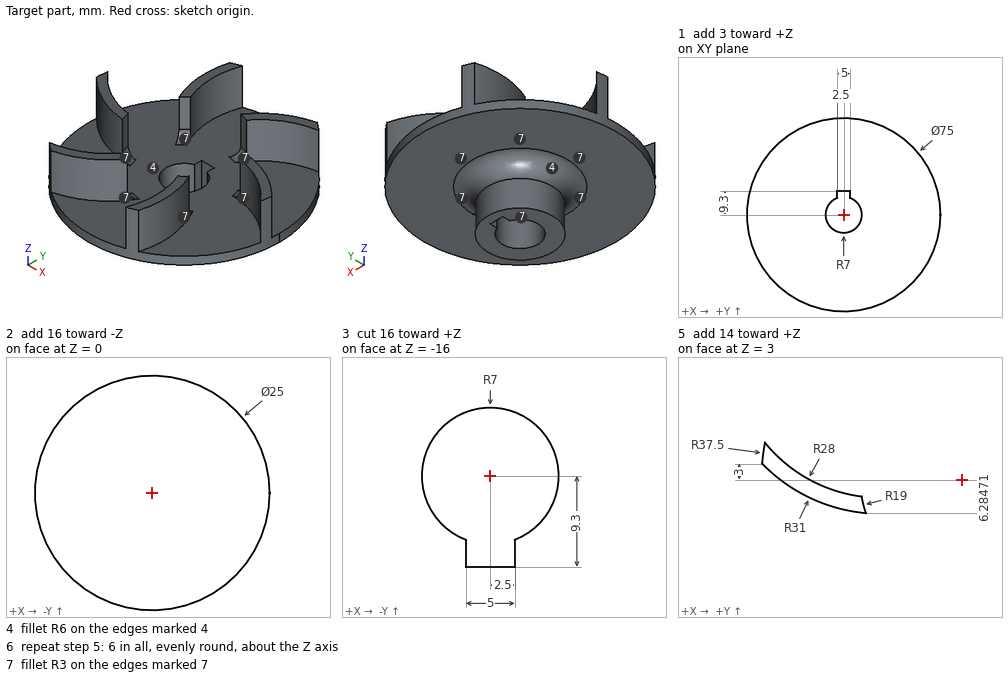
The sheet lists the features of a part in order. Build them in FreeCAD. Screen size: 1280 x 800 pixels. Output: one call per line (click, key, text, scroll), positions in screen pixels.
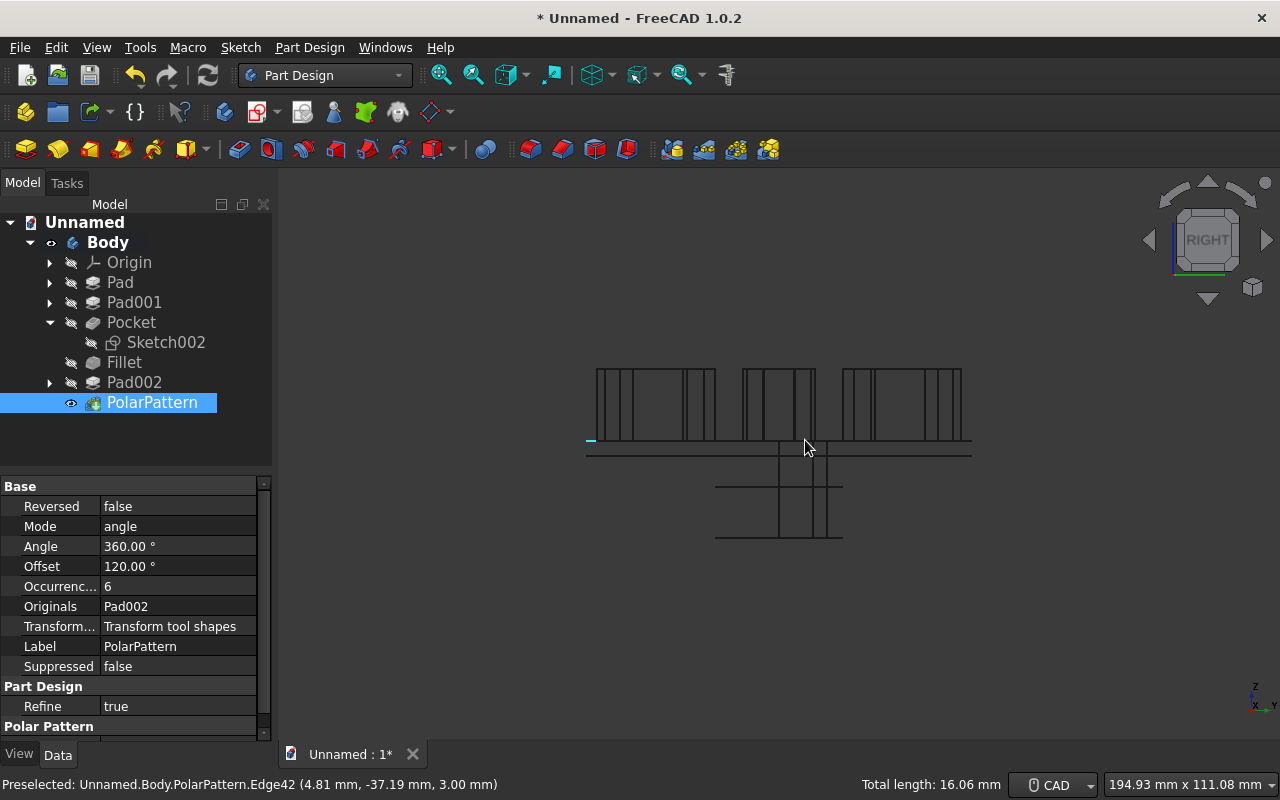
scroll(873, 440, up, 5)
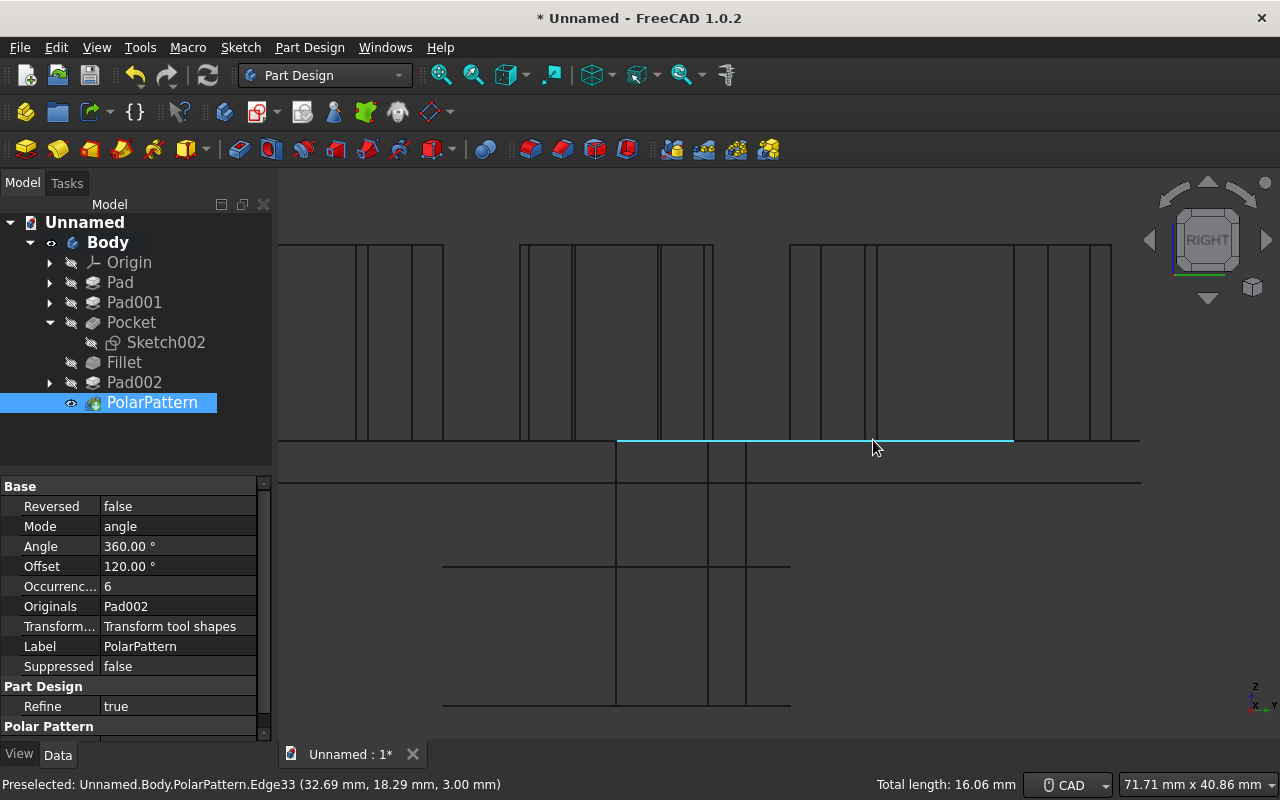
key(v)
key(f)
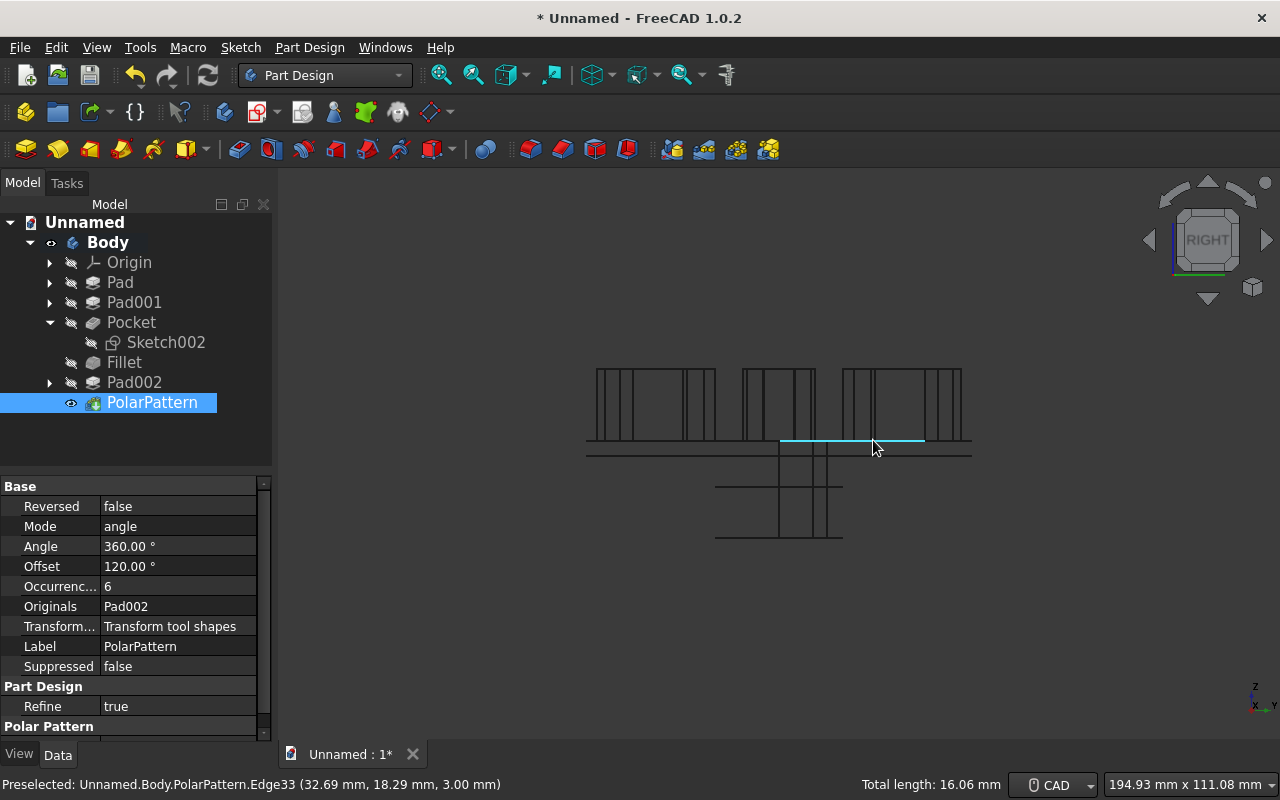
key(5)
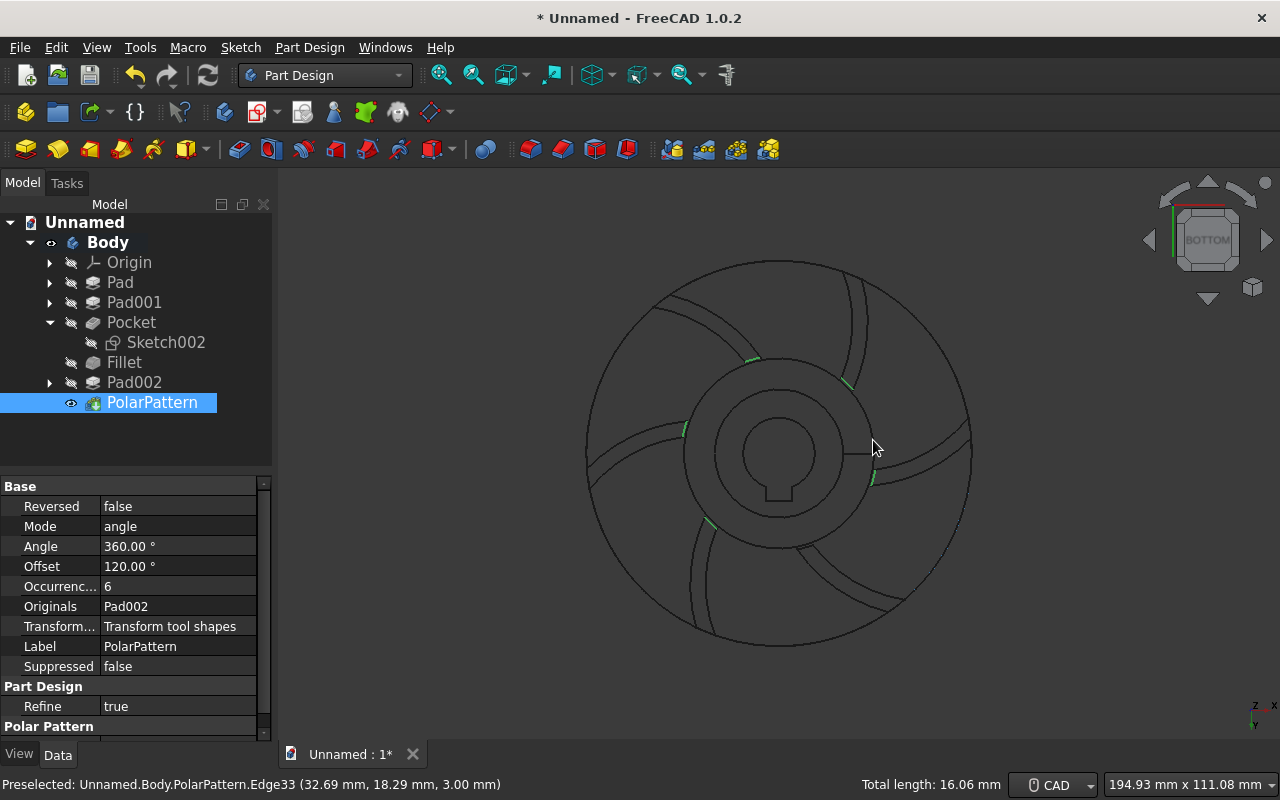
scroll(805, 547, up, 5)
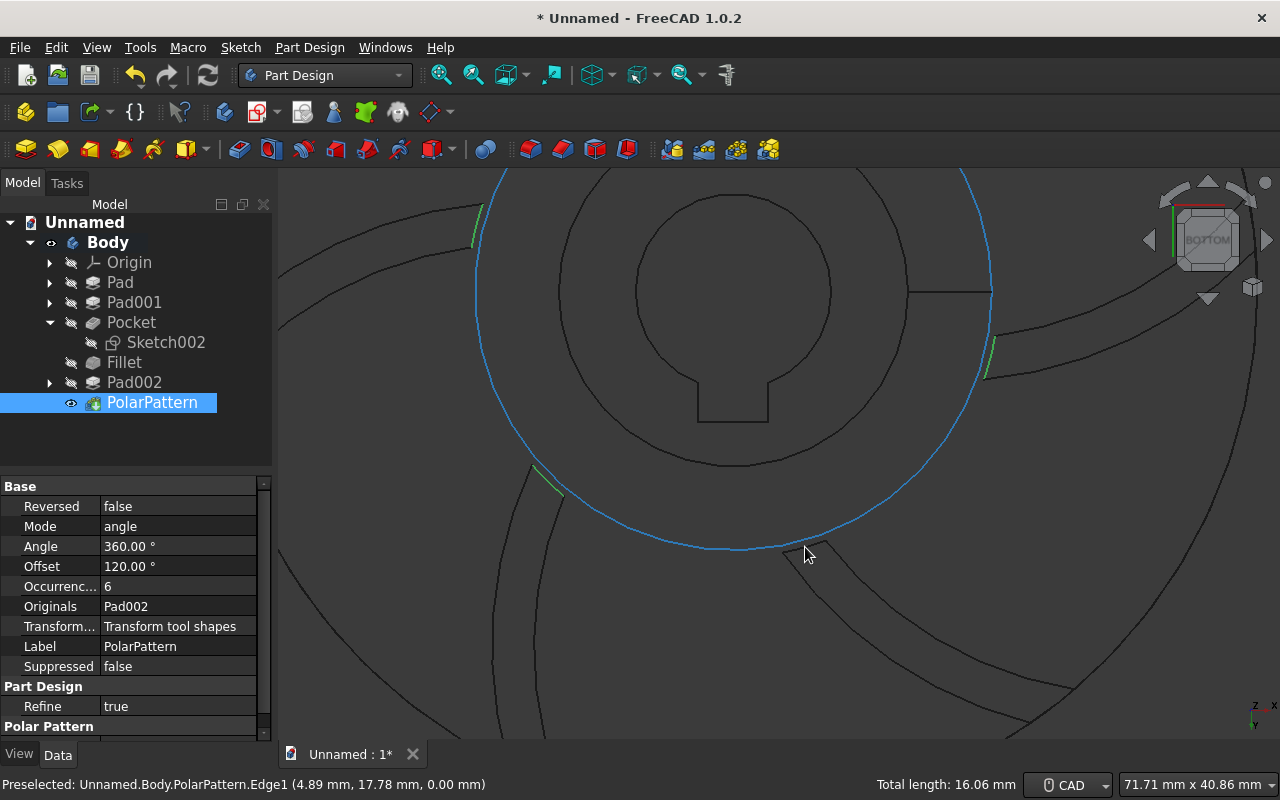
click(804, 546, ctrl)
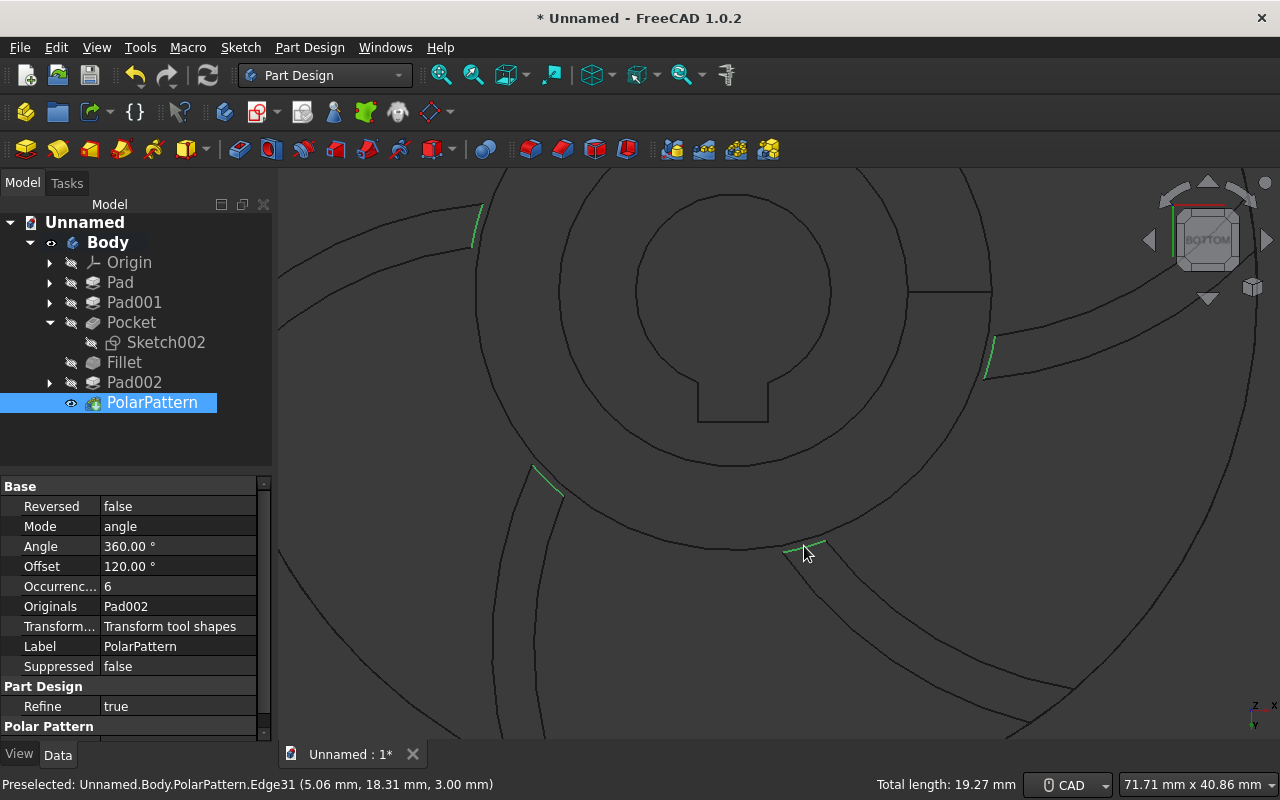
key(v)
key(1)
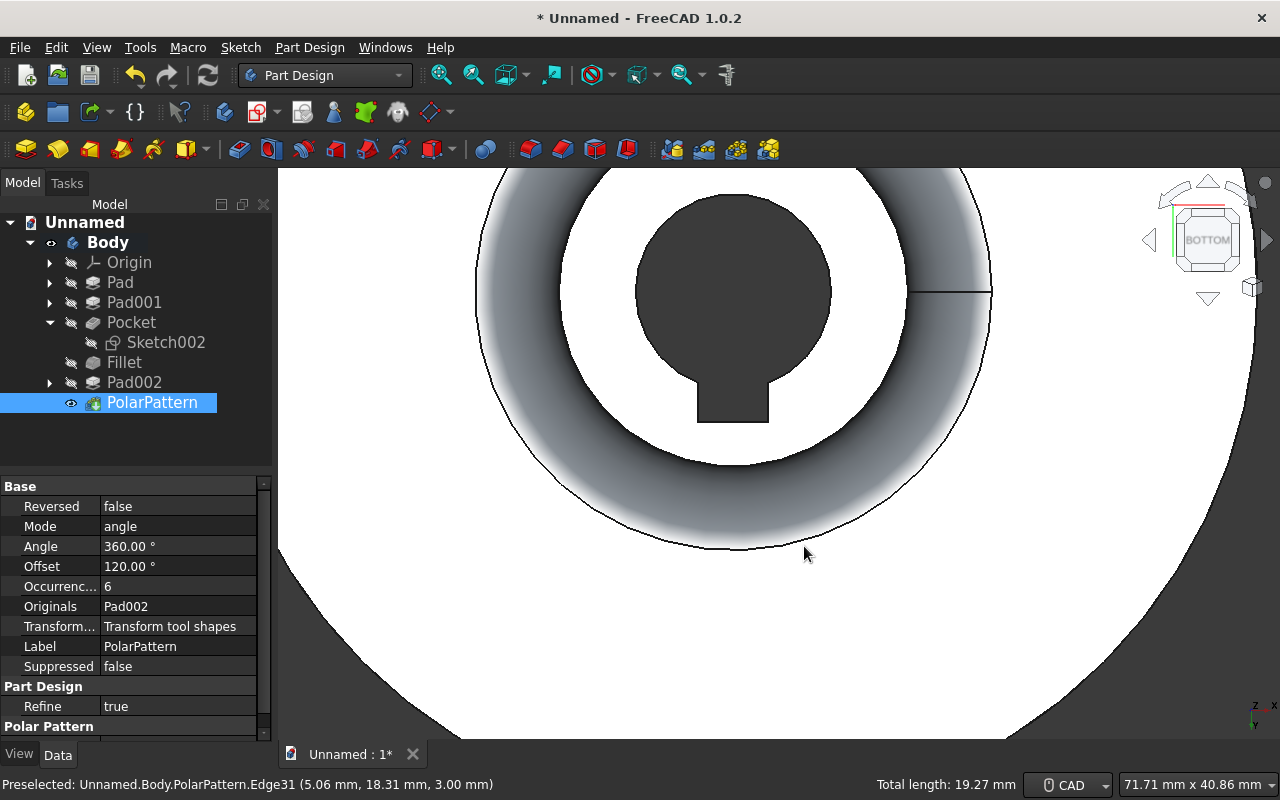
click(532, 150)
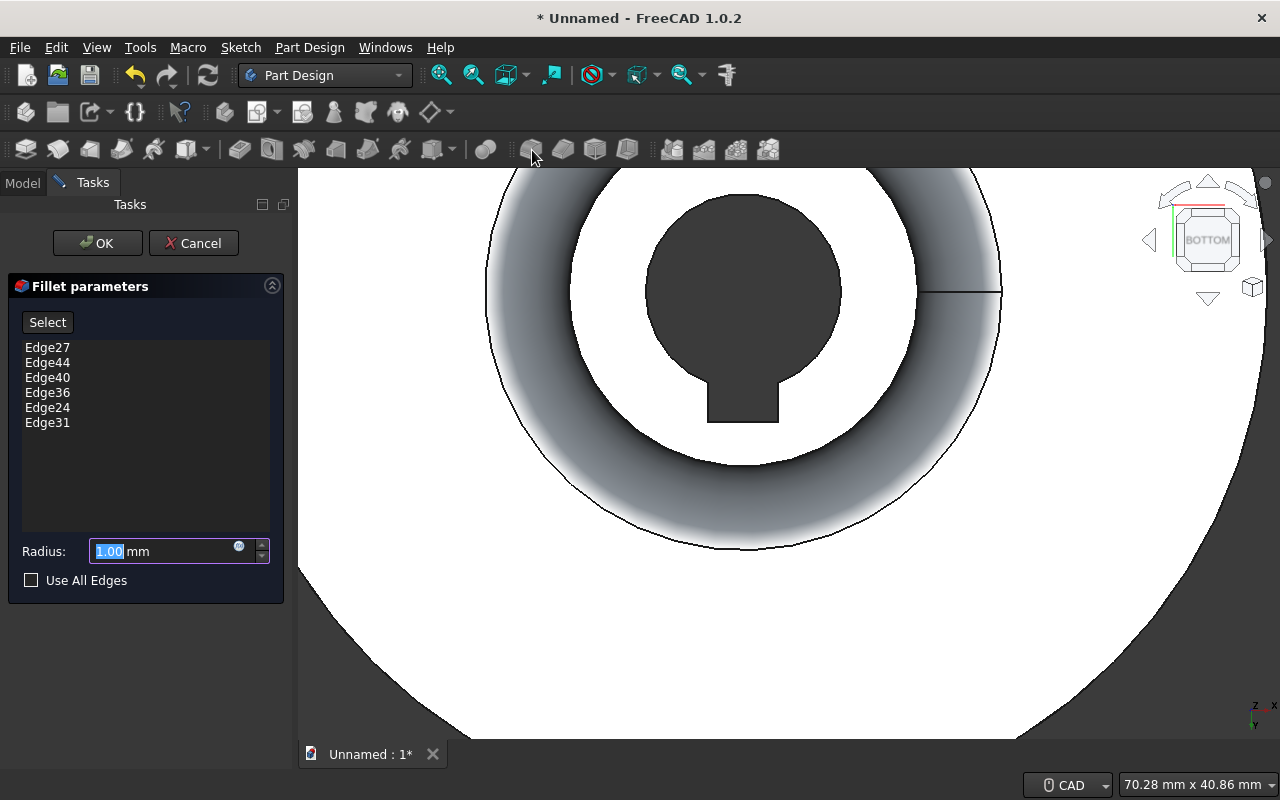
text(3)
key(Tab)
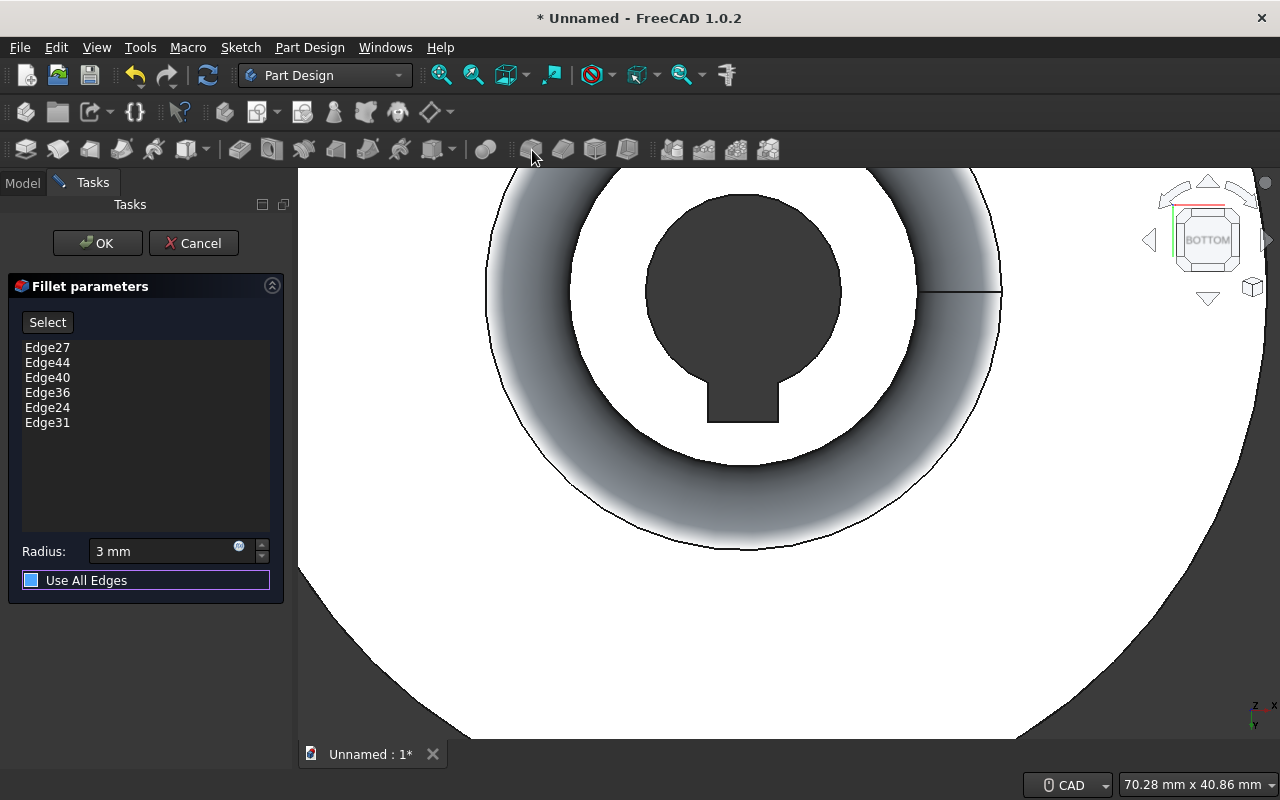
click(98, 243)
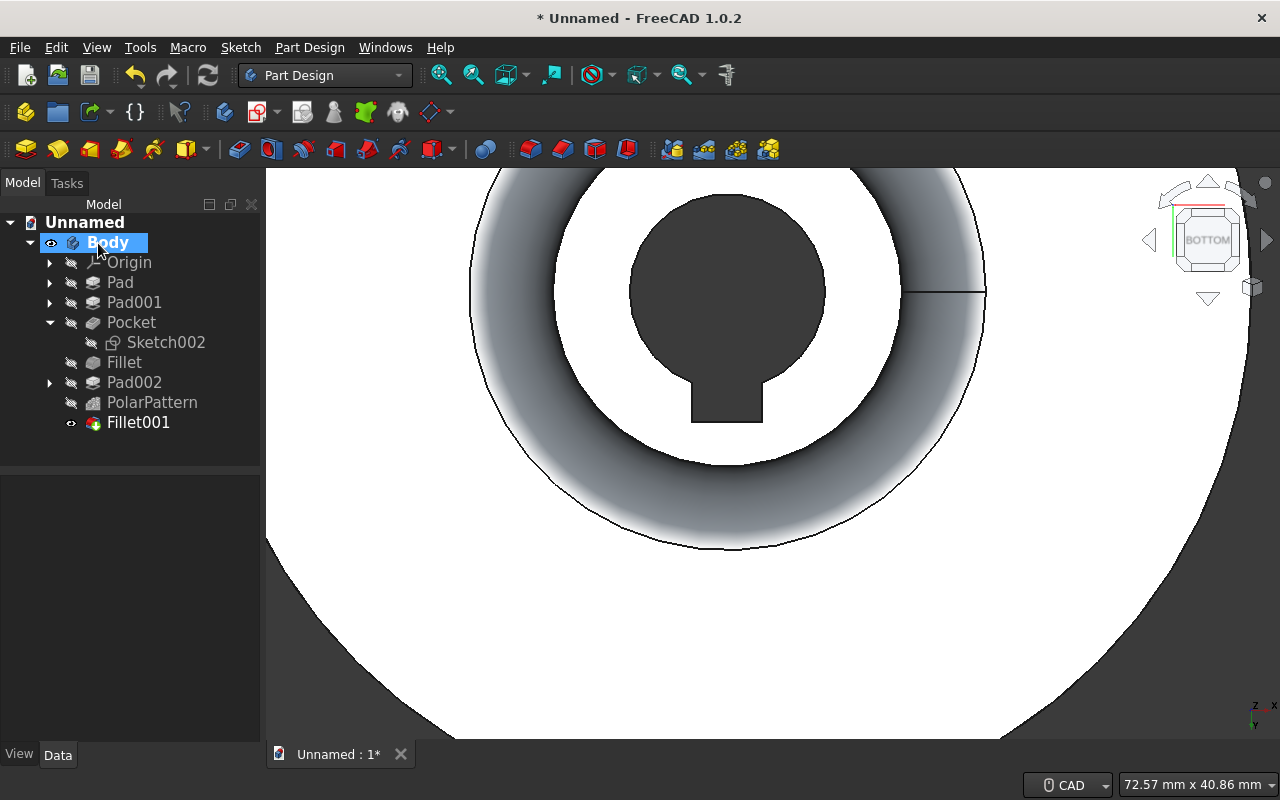
key(0)